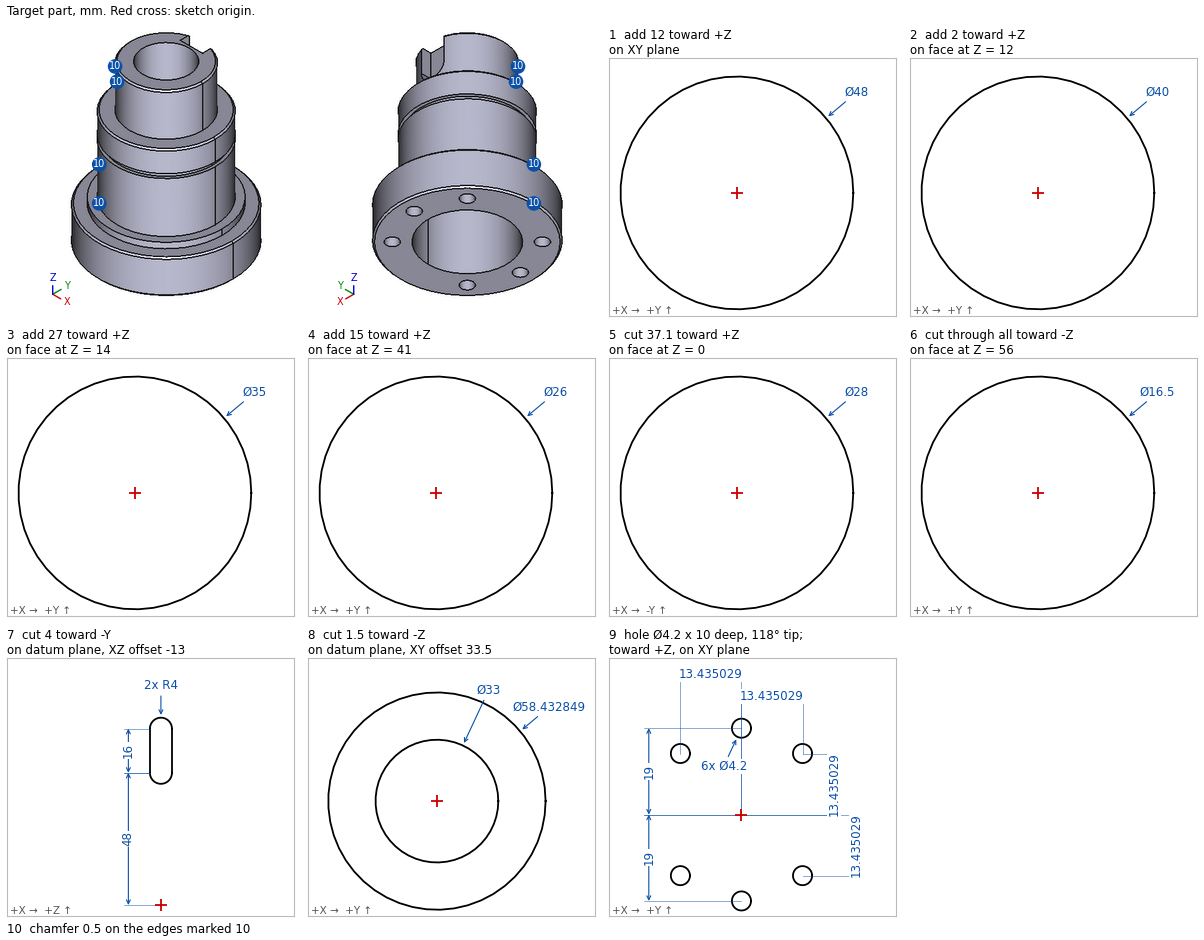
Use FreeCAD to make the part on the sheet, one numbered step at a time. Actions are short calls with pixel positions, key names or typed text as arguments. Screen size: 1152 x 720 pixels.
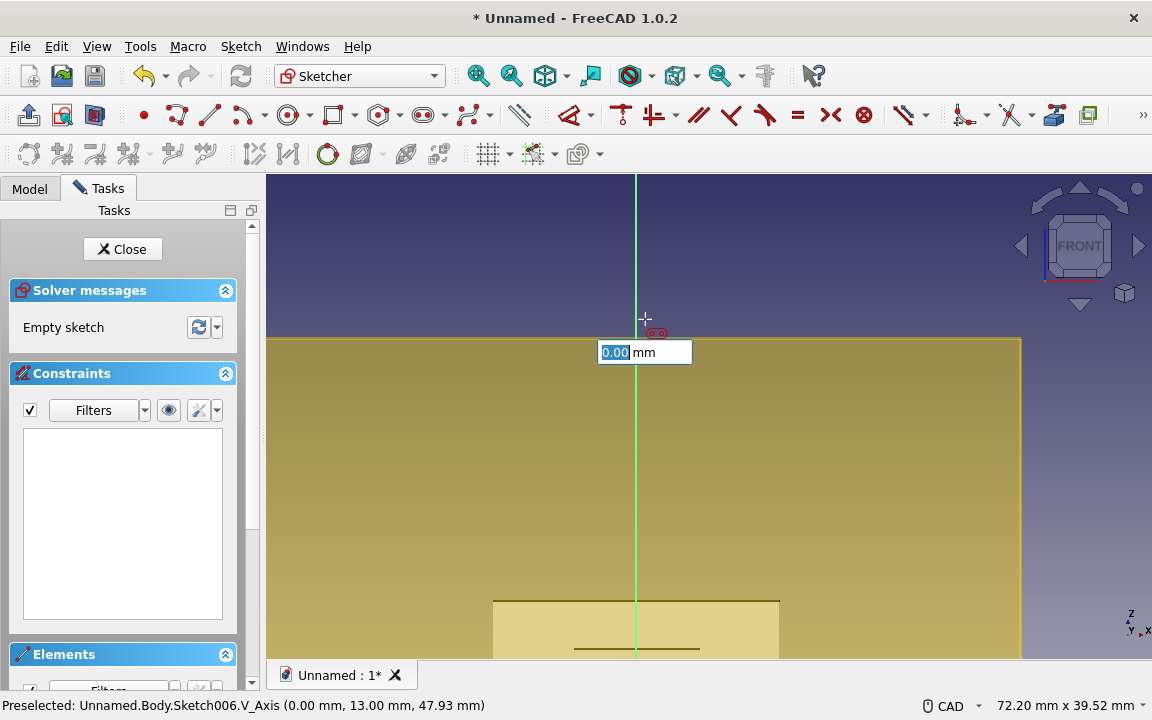
click(685, 417)
key(Escape)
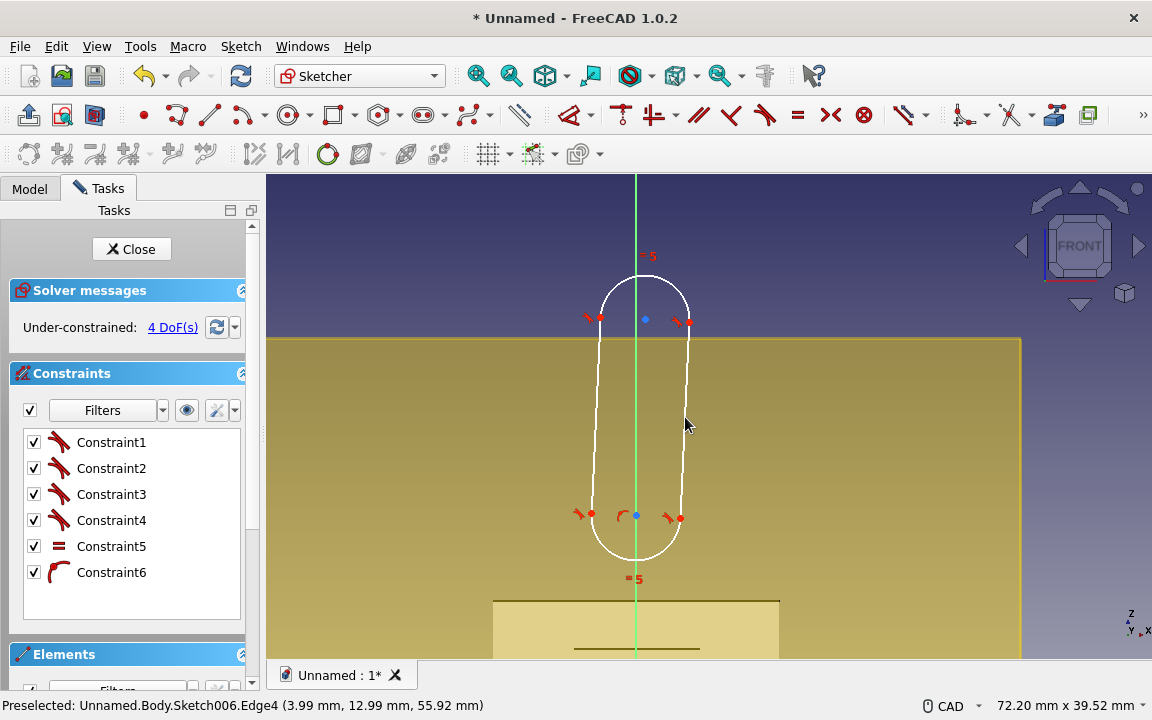
click(594, 455)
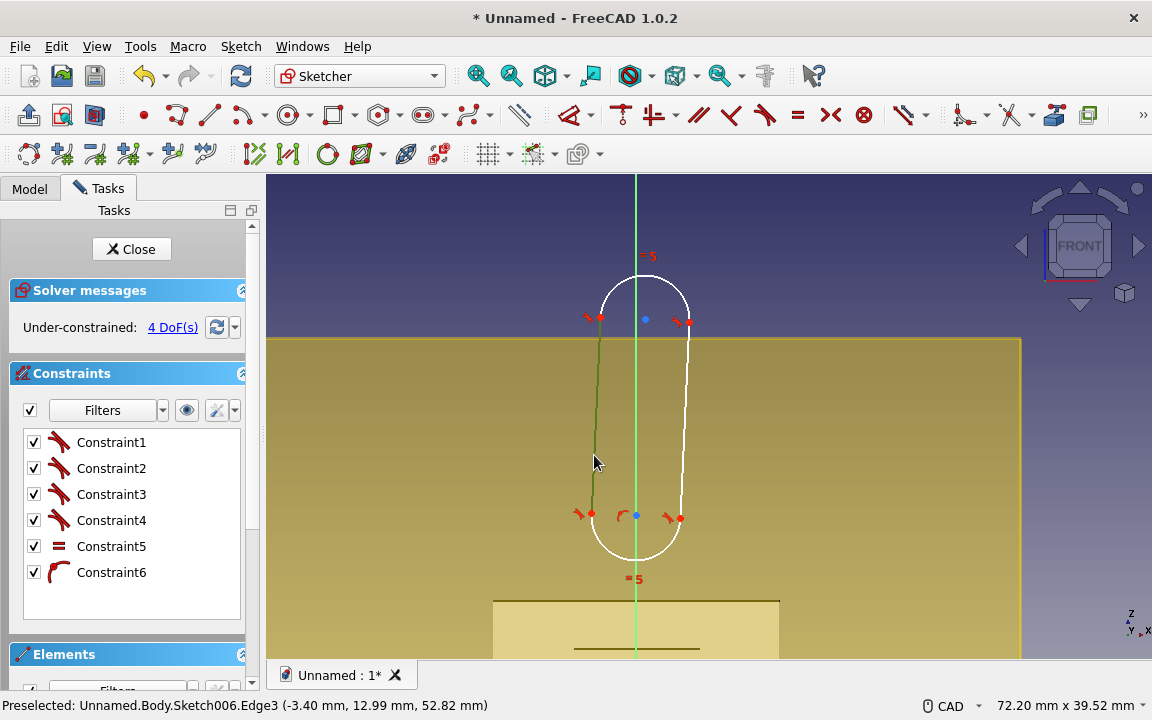
key(v)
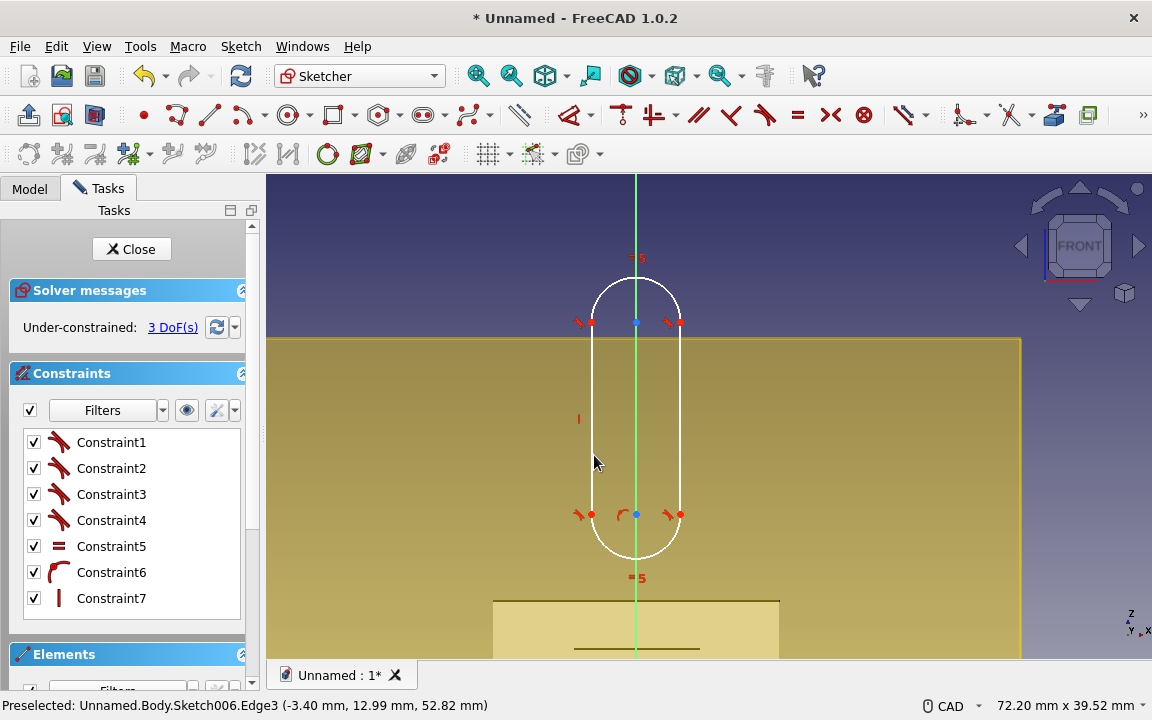
click(610, 550)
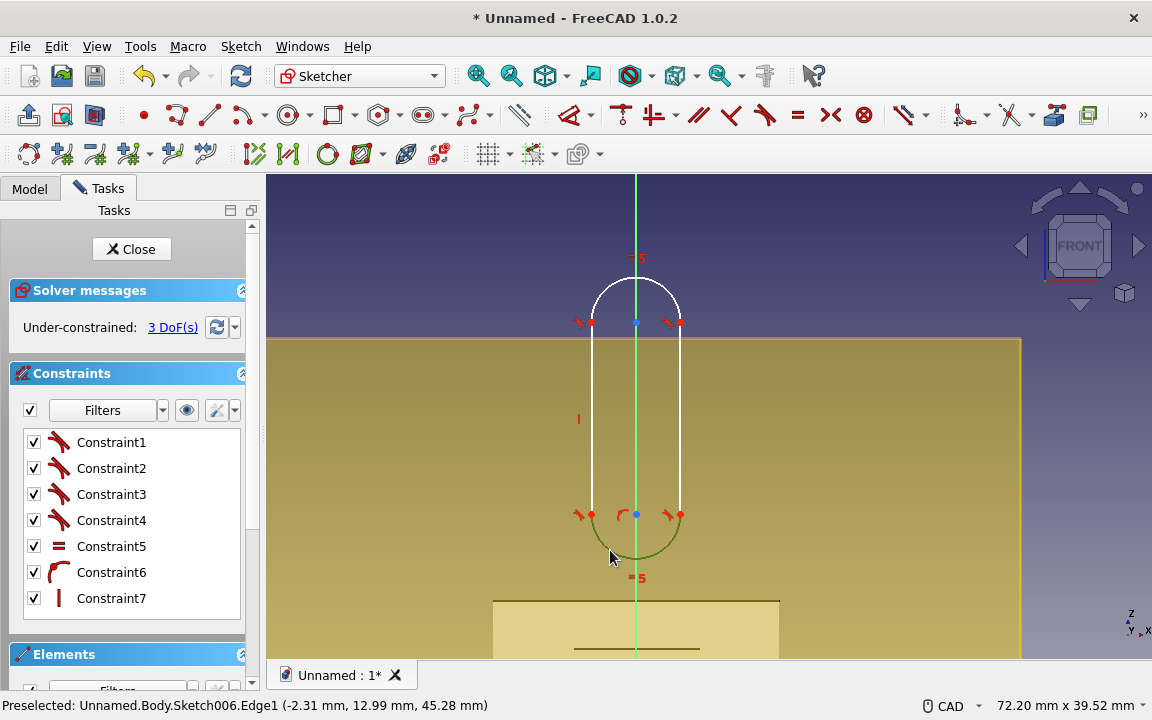
key(k)
key(r)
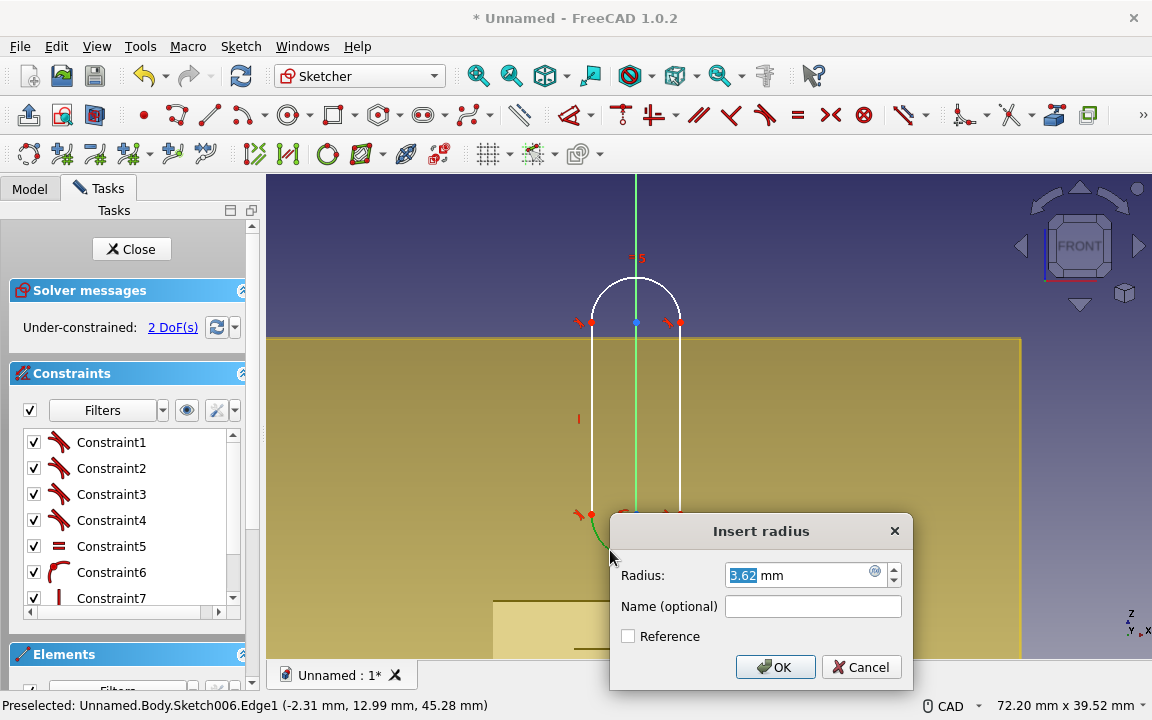
text(4)
key(Return)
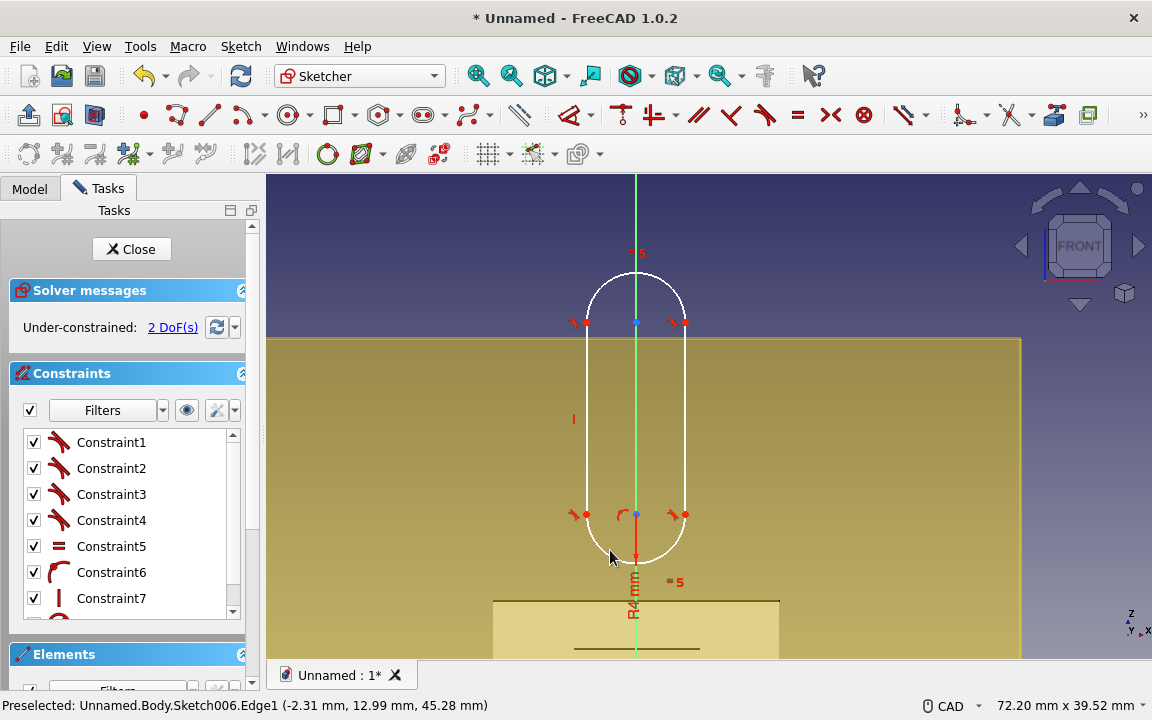
click(587, 457)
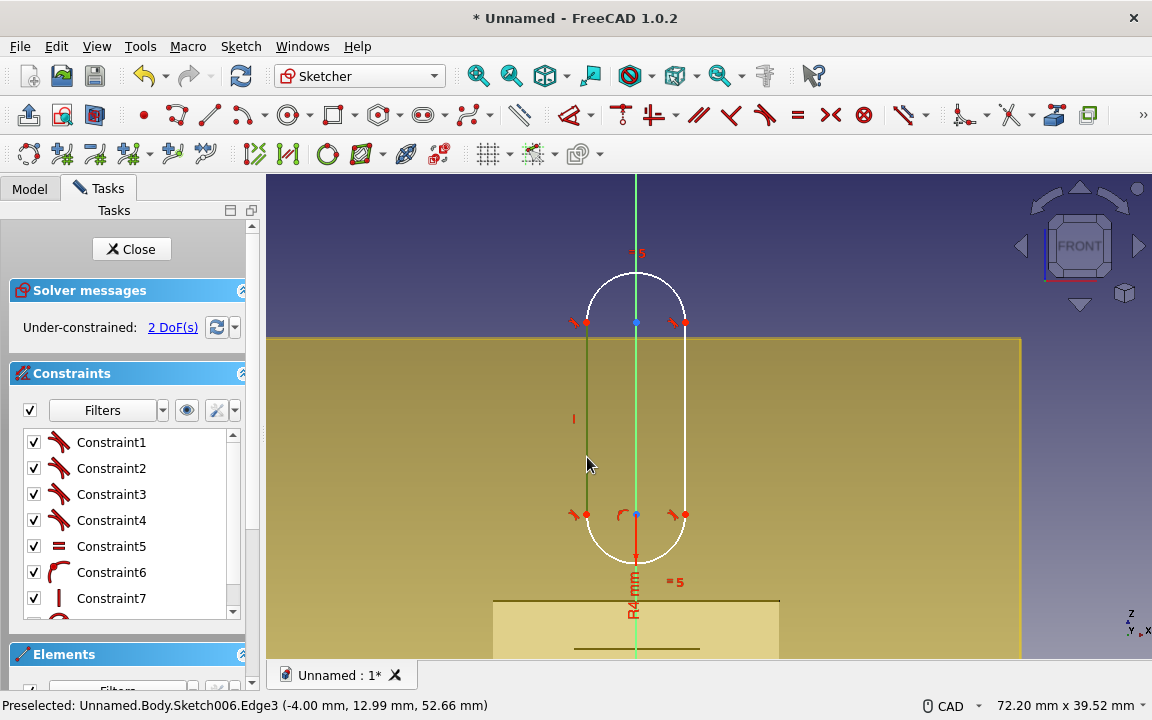
click(590, 116)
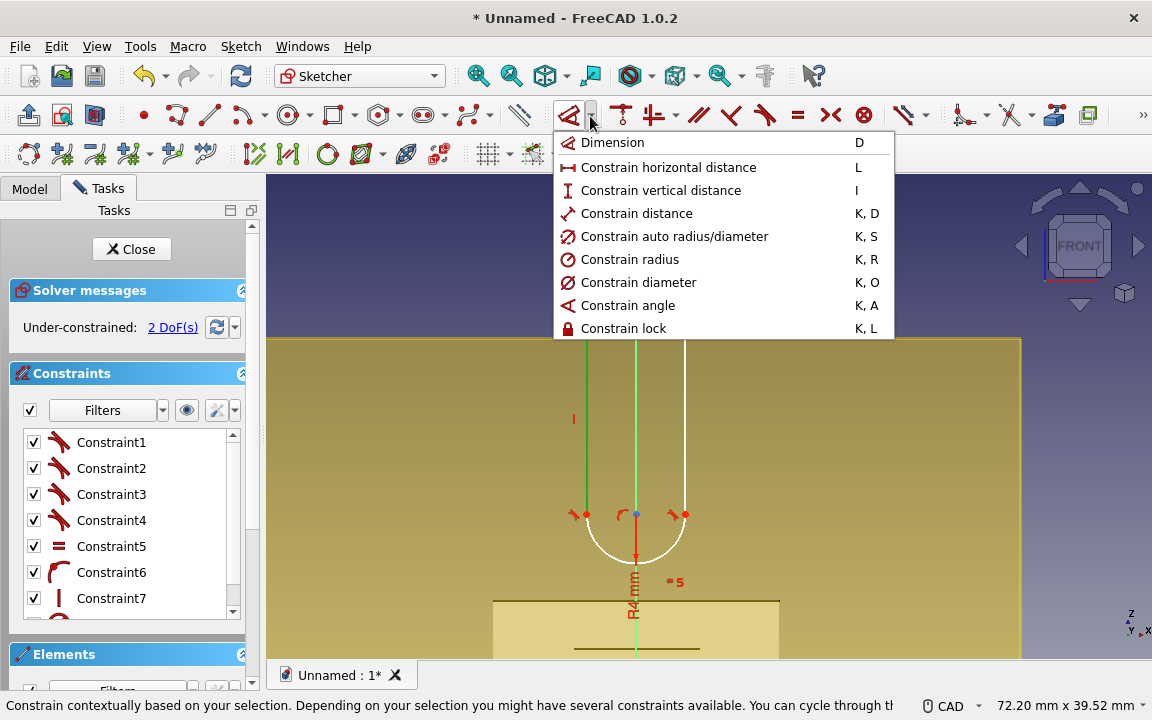
click(724, 190)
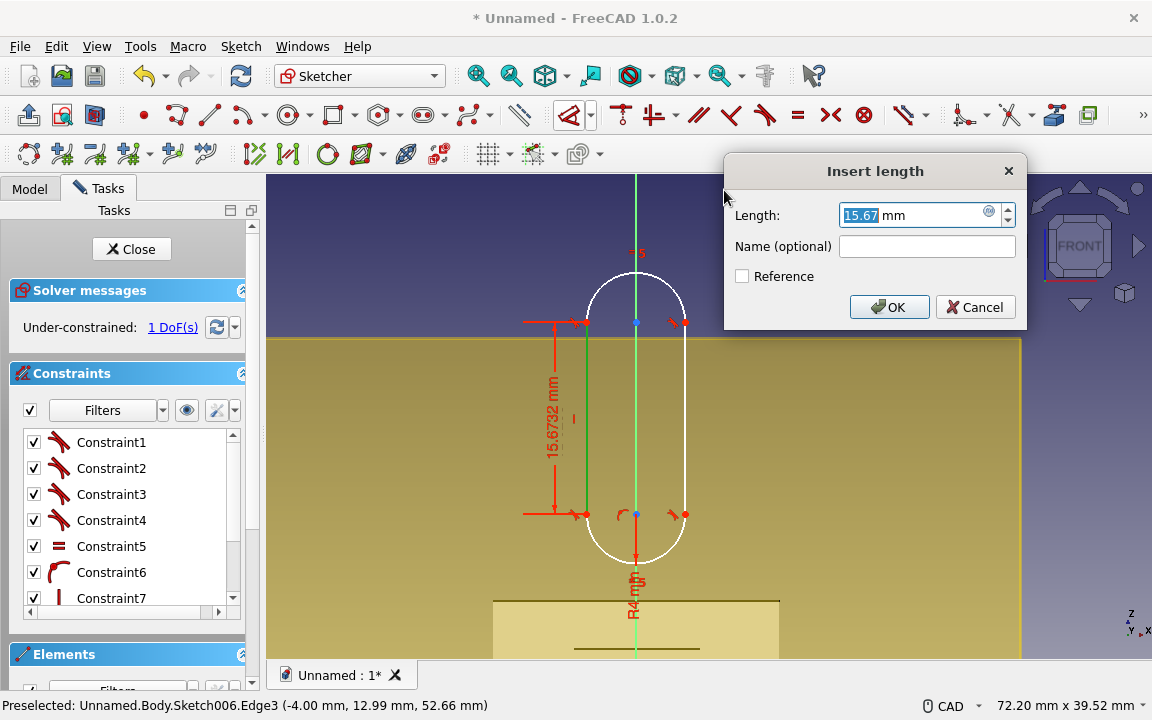
text(16)
key(Return)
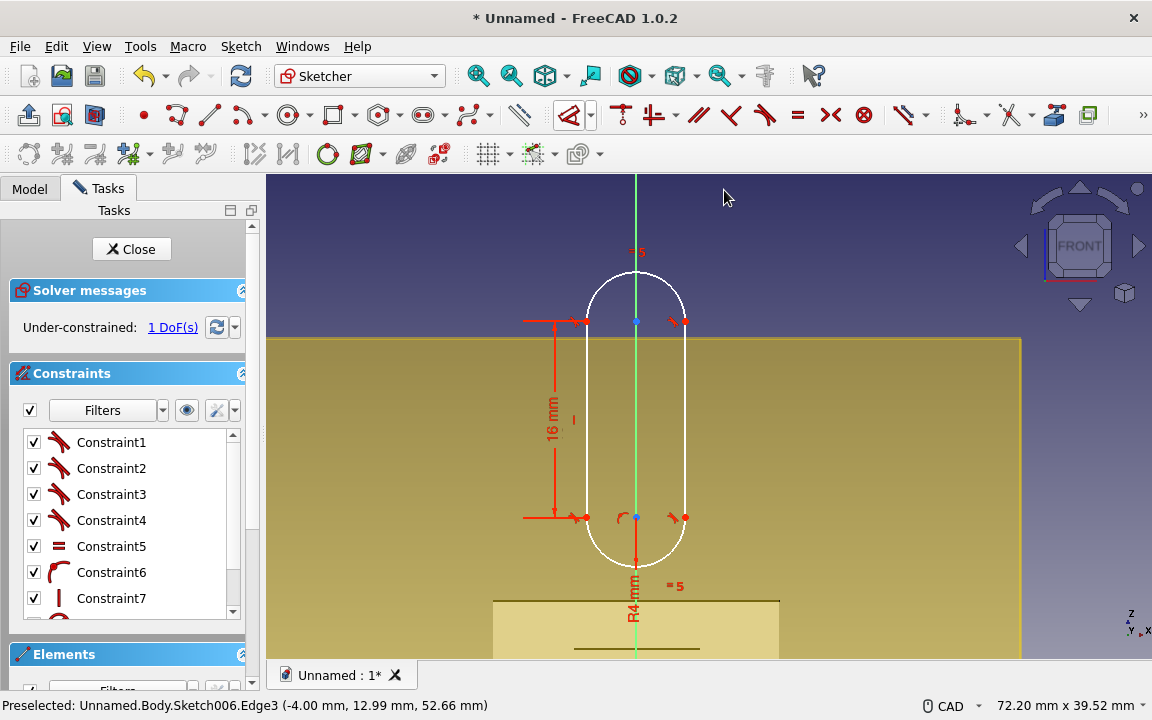
click(587, 518)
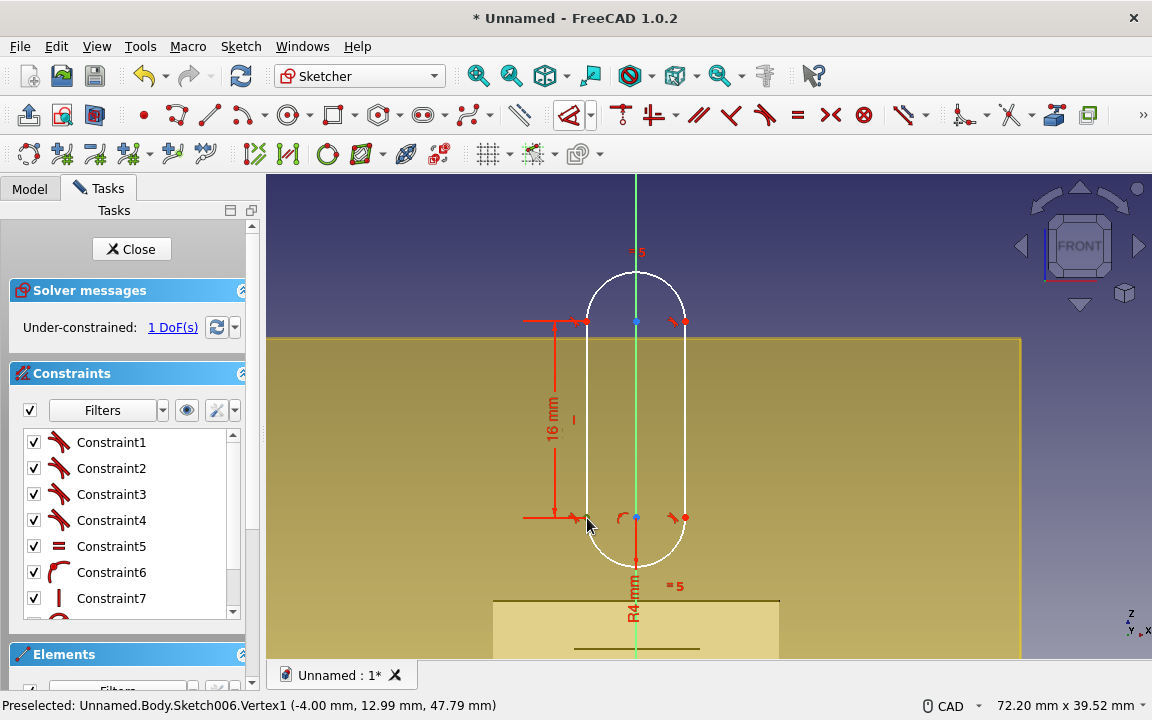
key(i)